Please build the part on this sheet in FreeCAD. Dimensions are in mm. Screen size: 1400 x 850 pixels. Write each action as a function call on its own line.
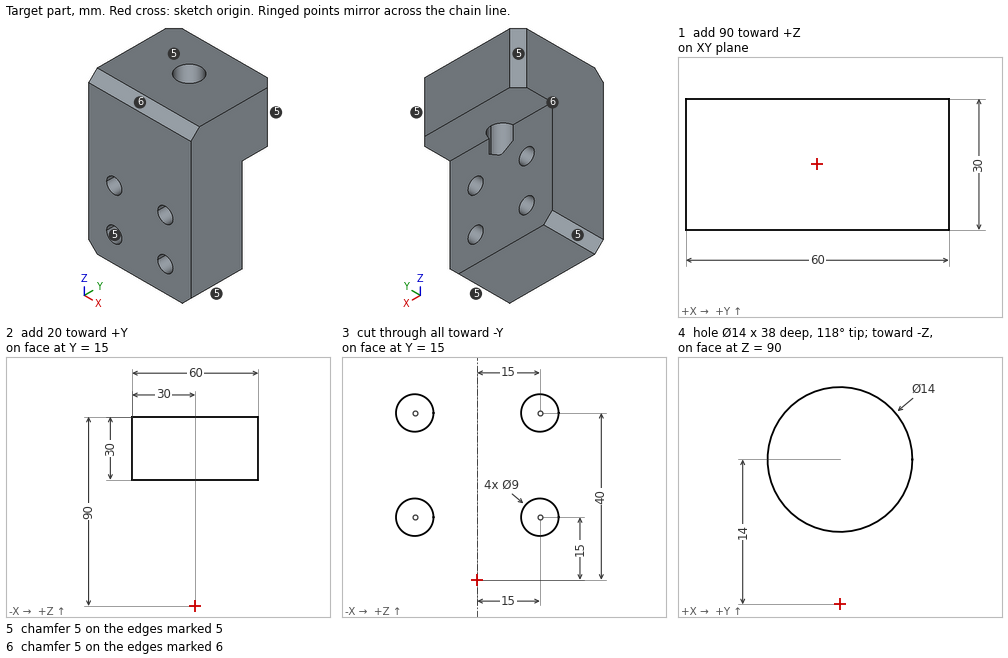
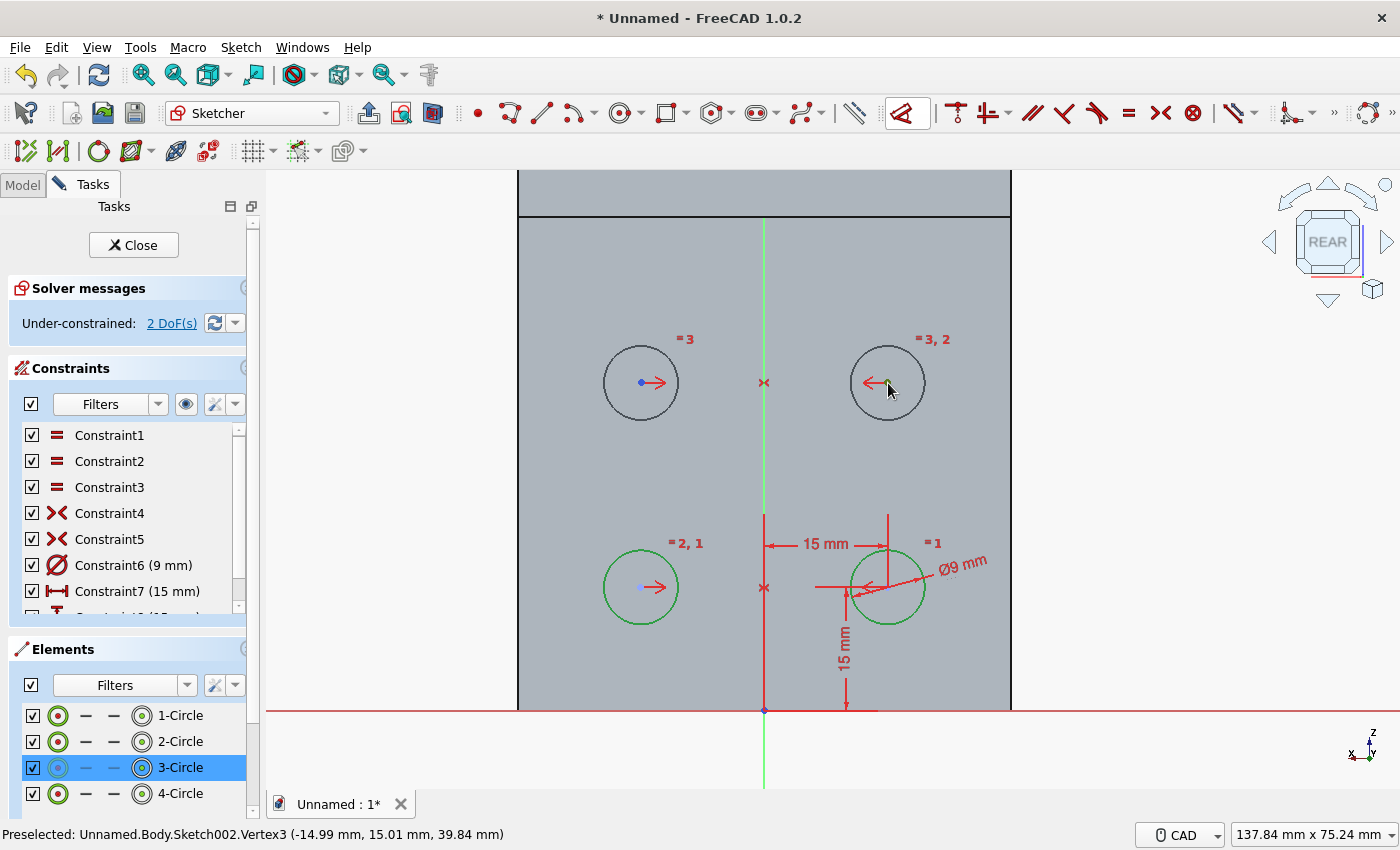
key(l)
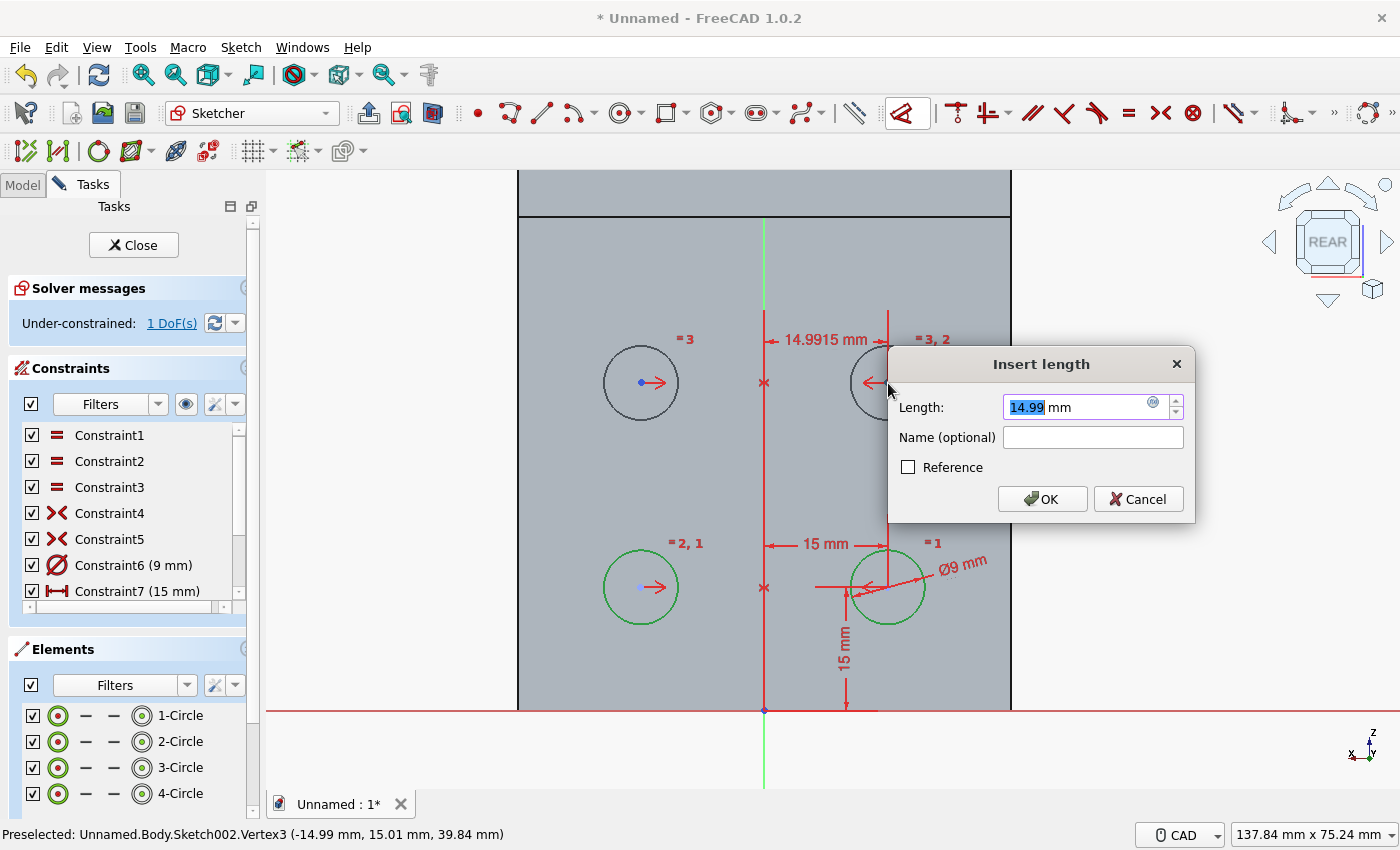
text(15)
key(Return)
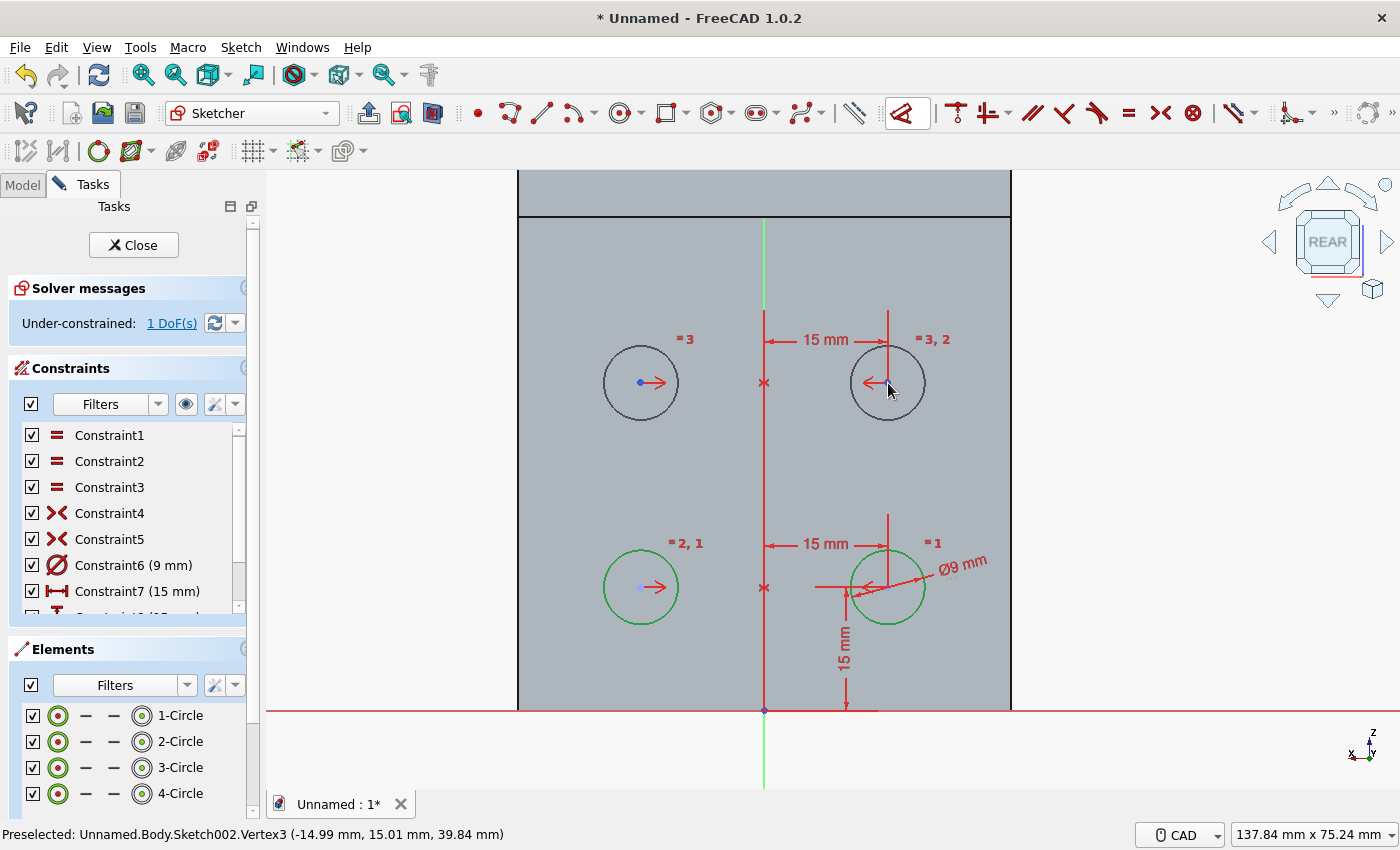
click(888, 383)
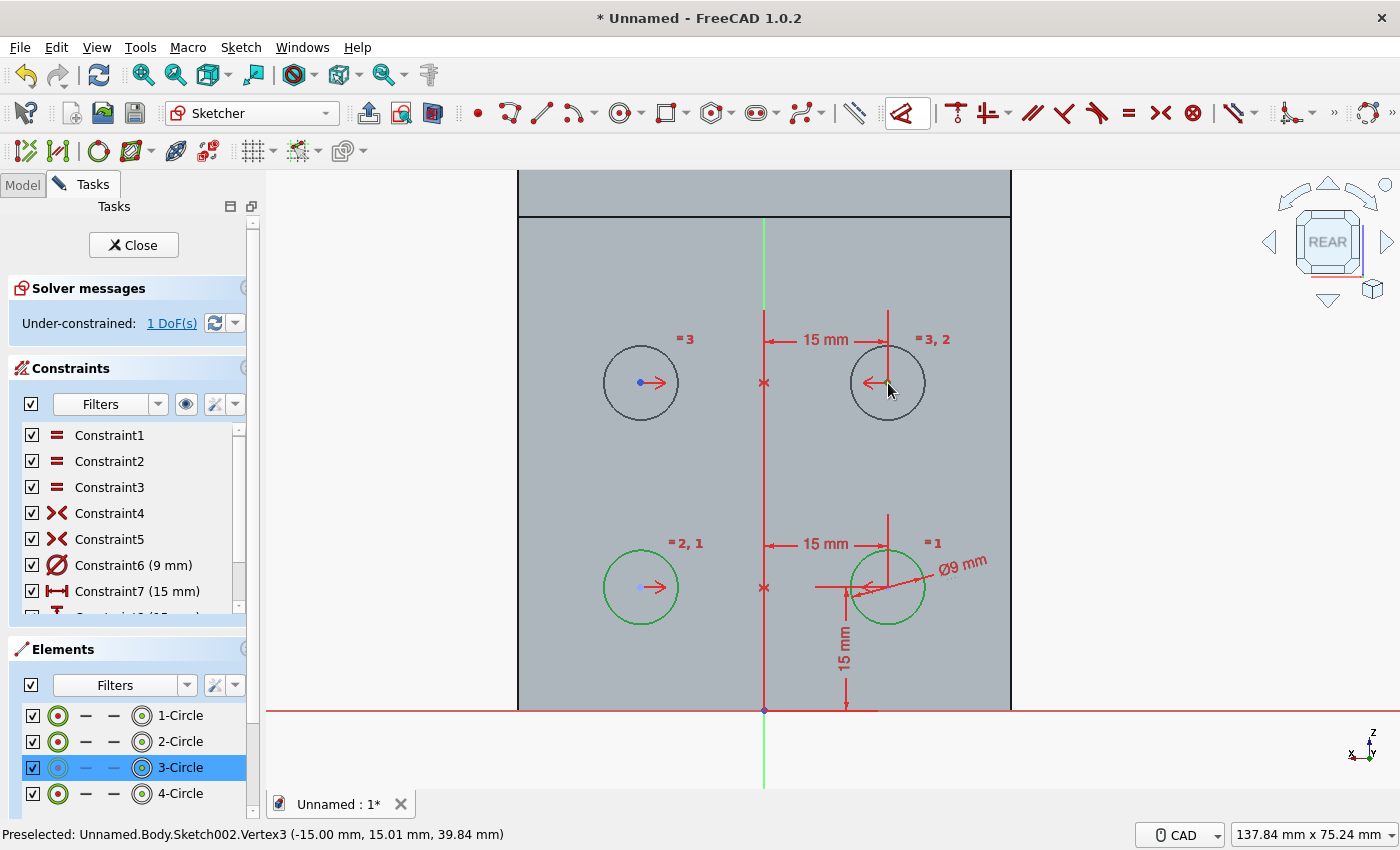
key(i)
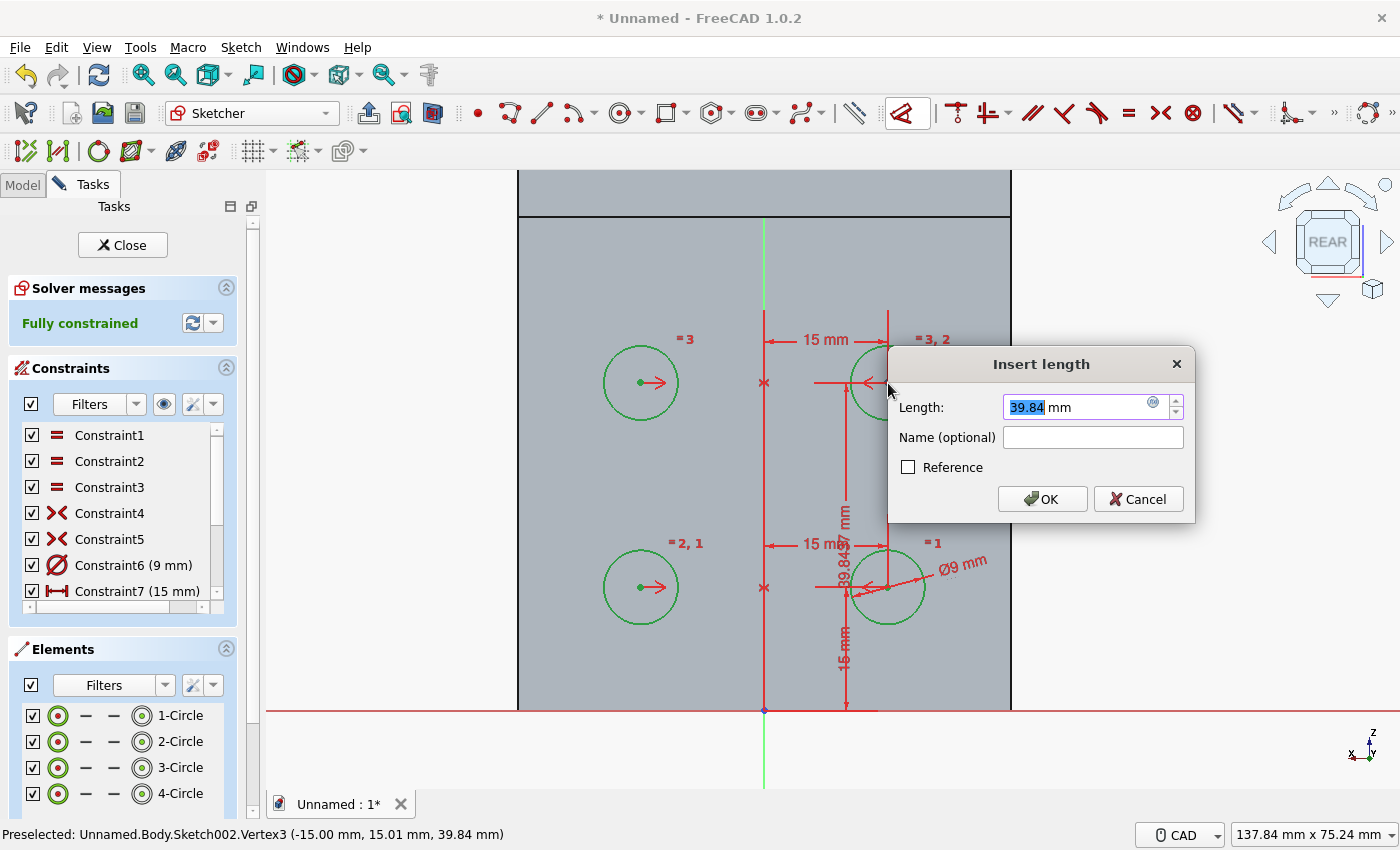
text(40)
key(Return)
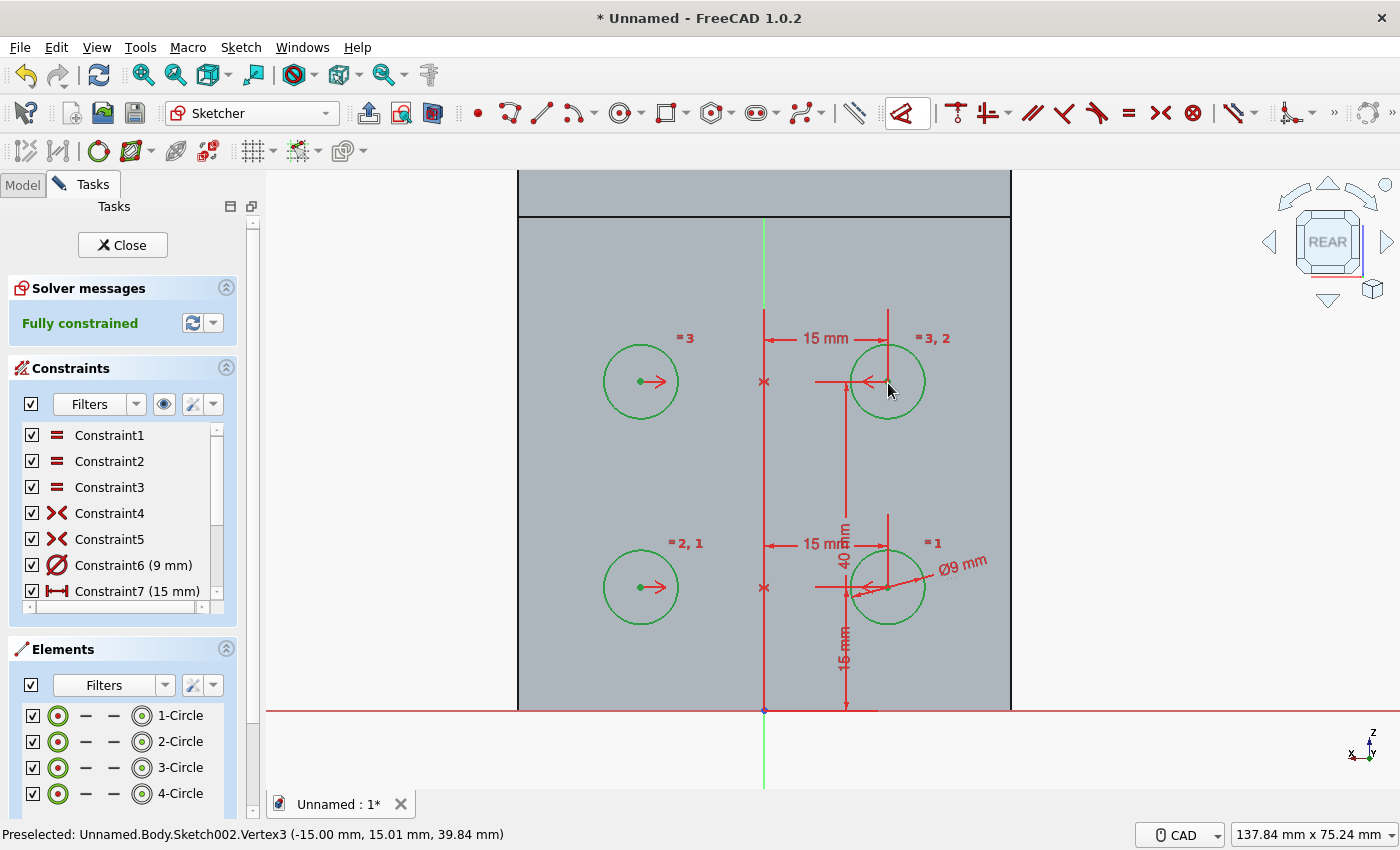
click(123, 245)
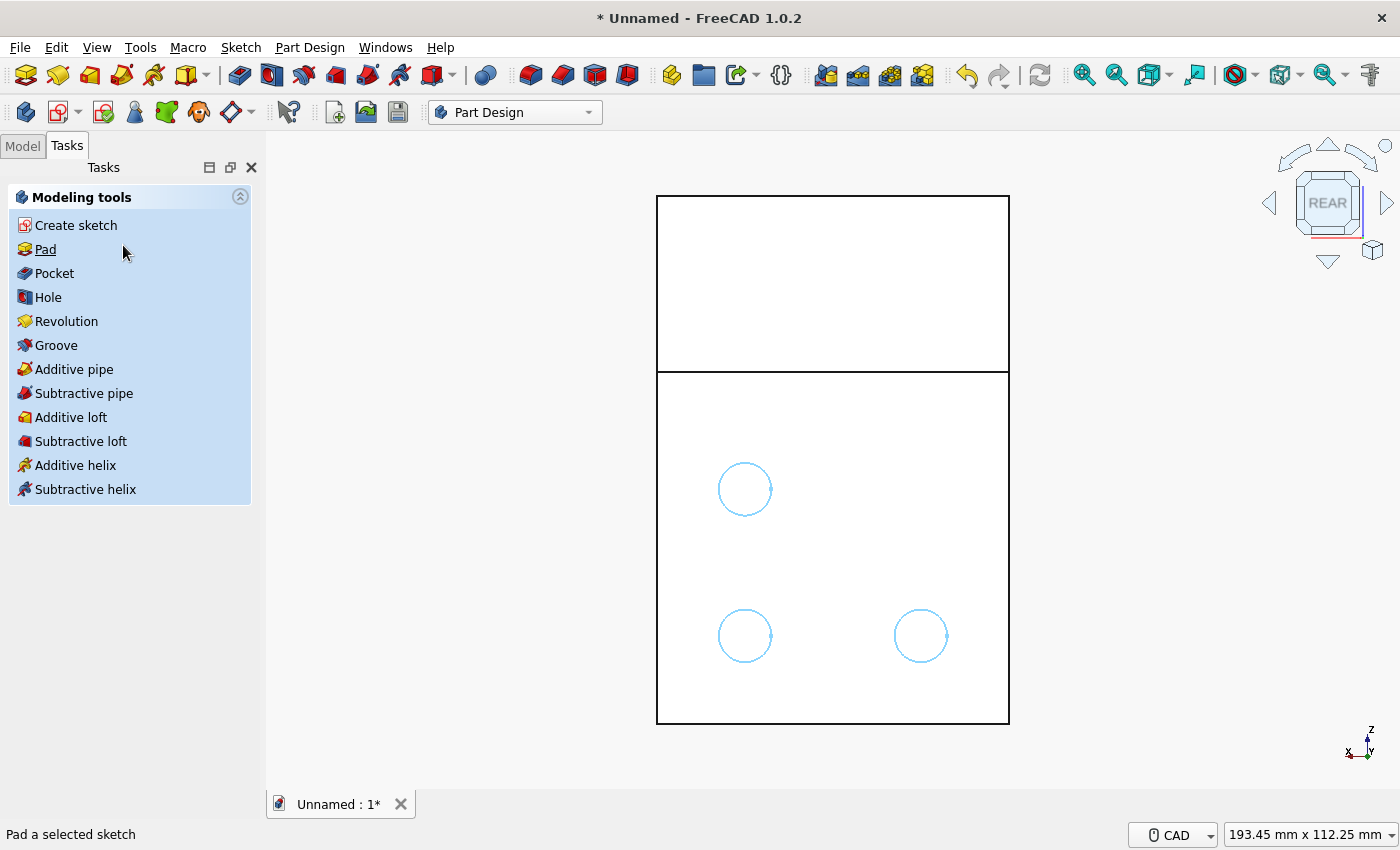
click(240, 76)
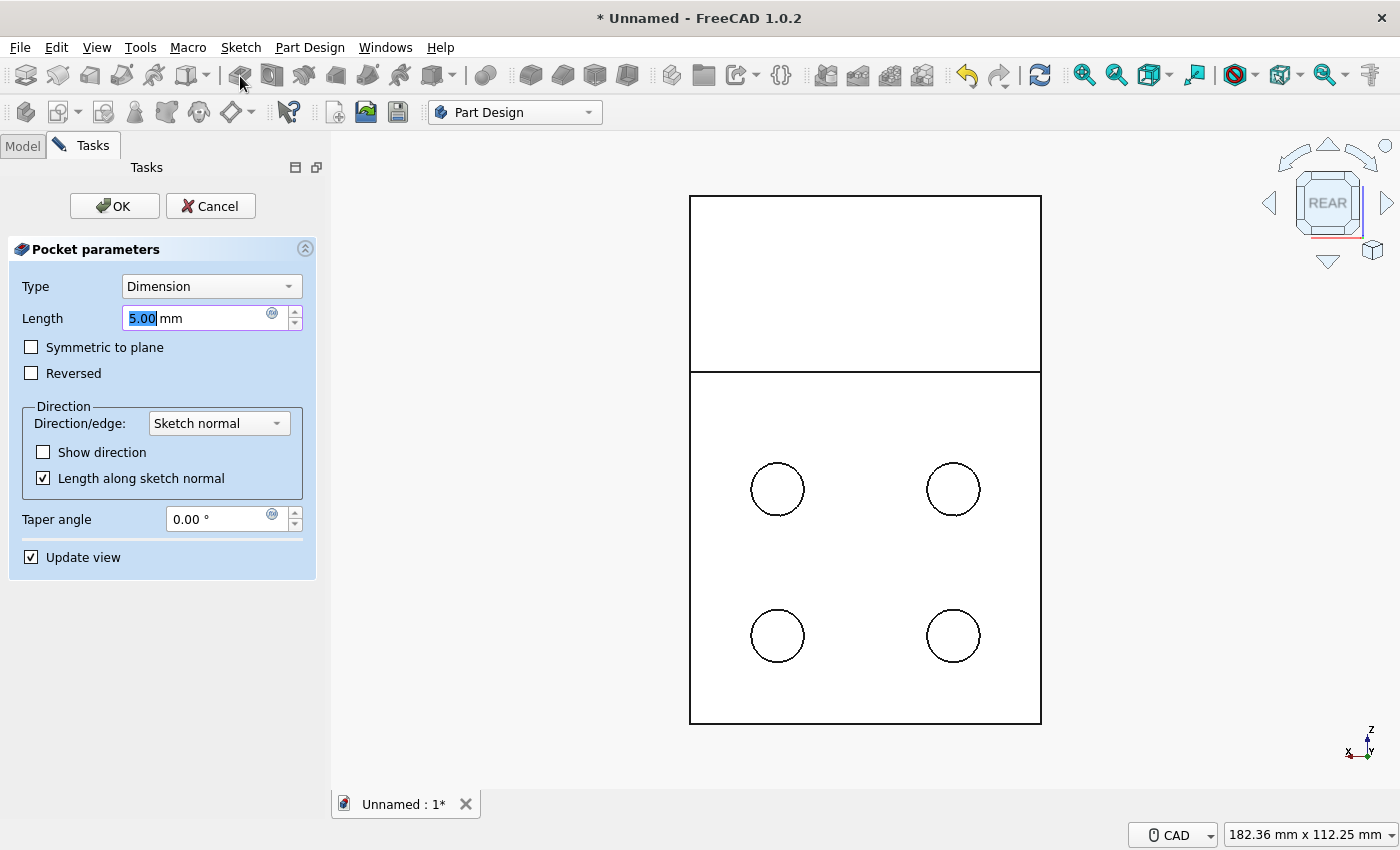
click(212, 286)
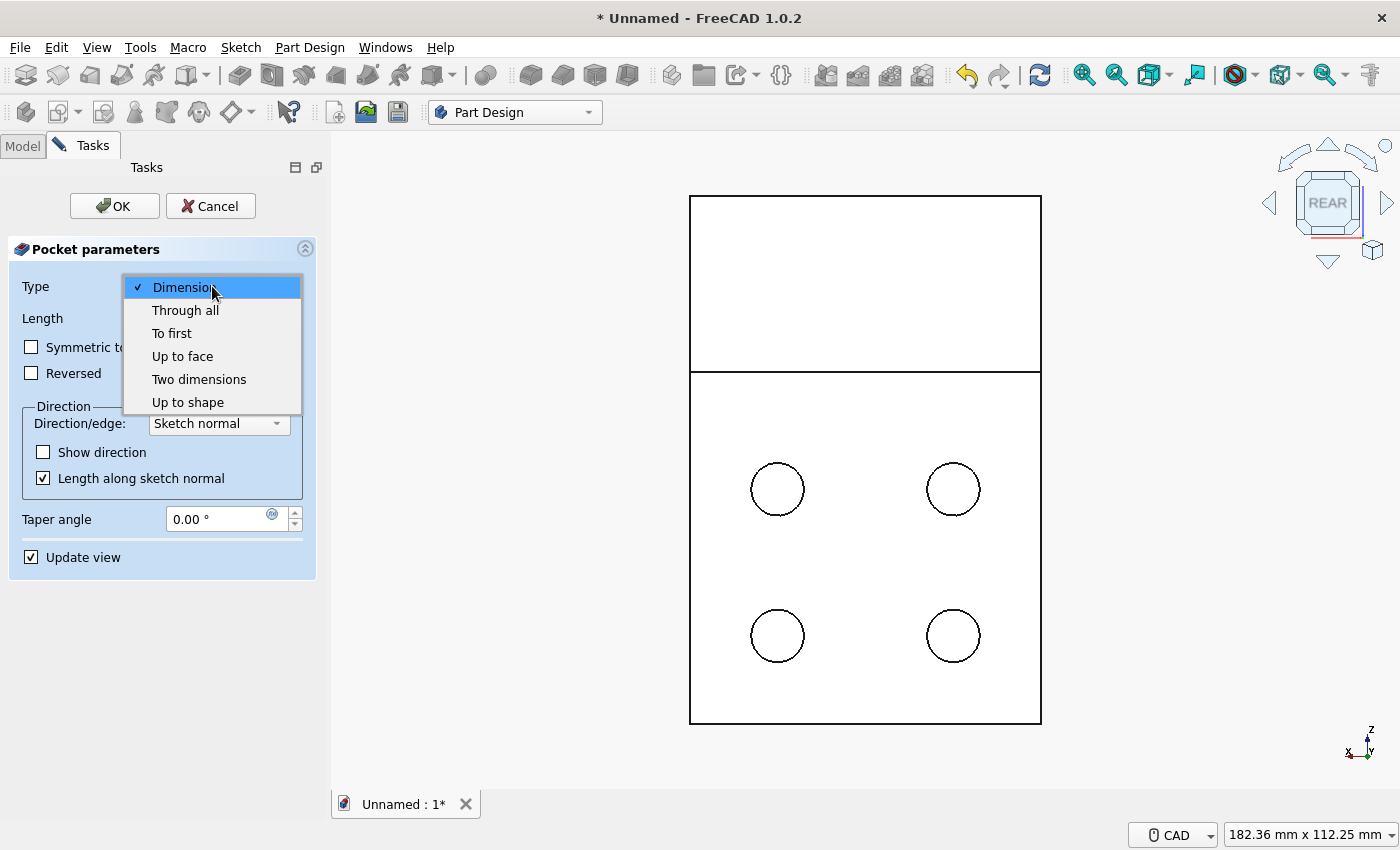
click(212, 310)